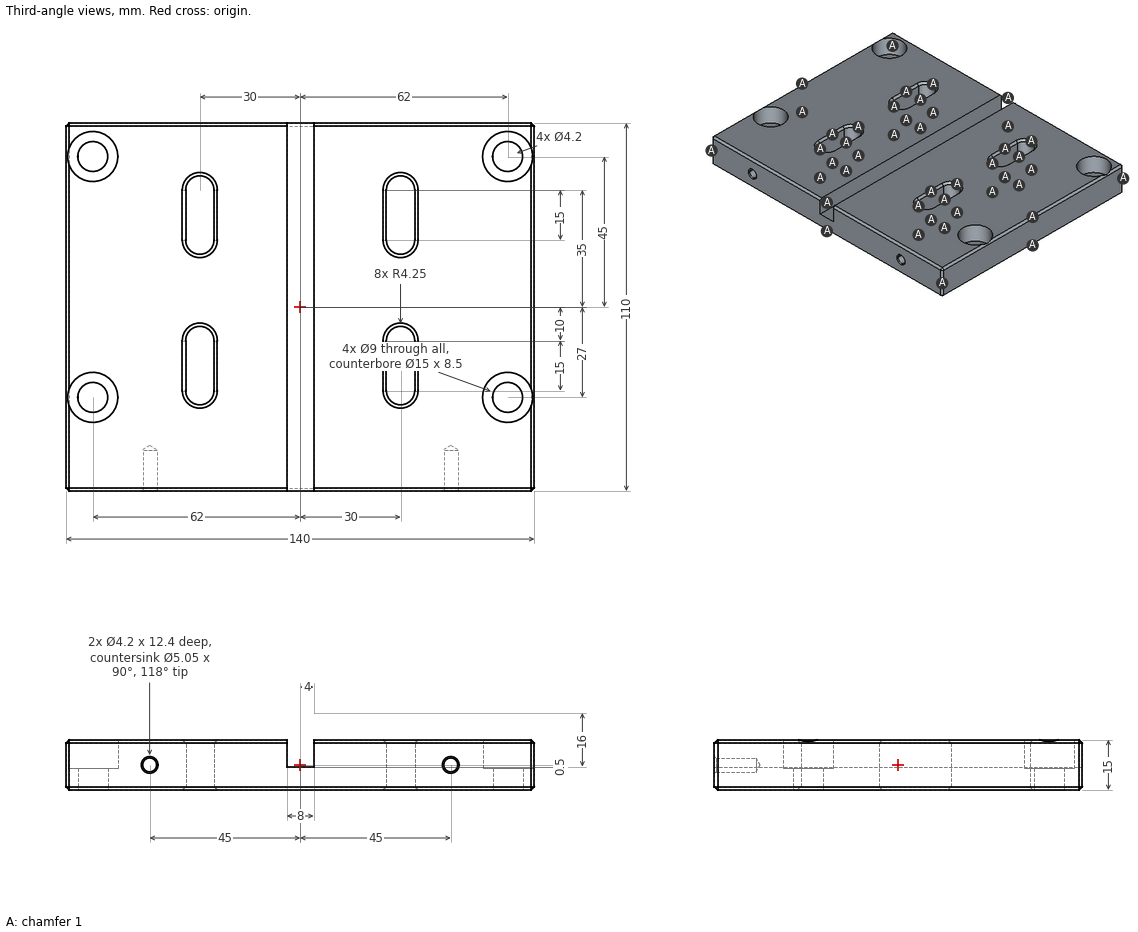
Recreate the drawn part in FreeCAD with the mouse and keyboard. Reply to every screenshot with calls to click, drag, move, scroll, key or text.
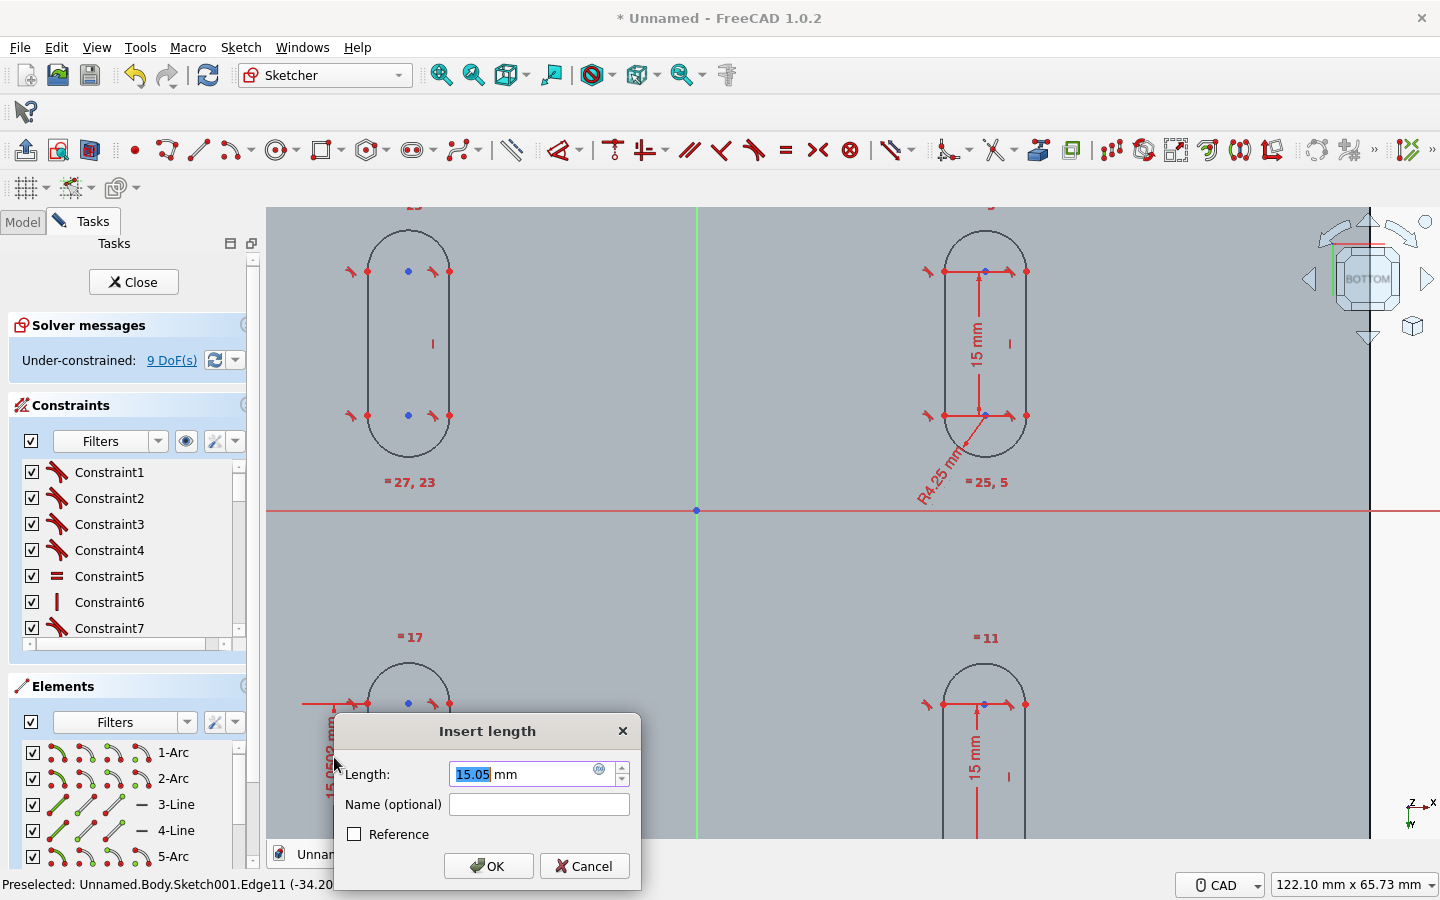
text(15)
key(Return)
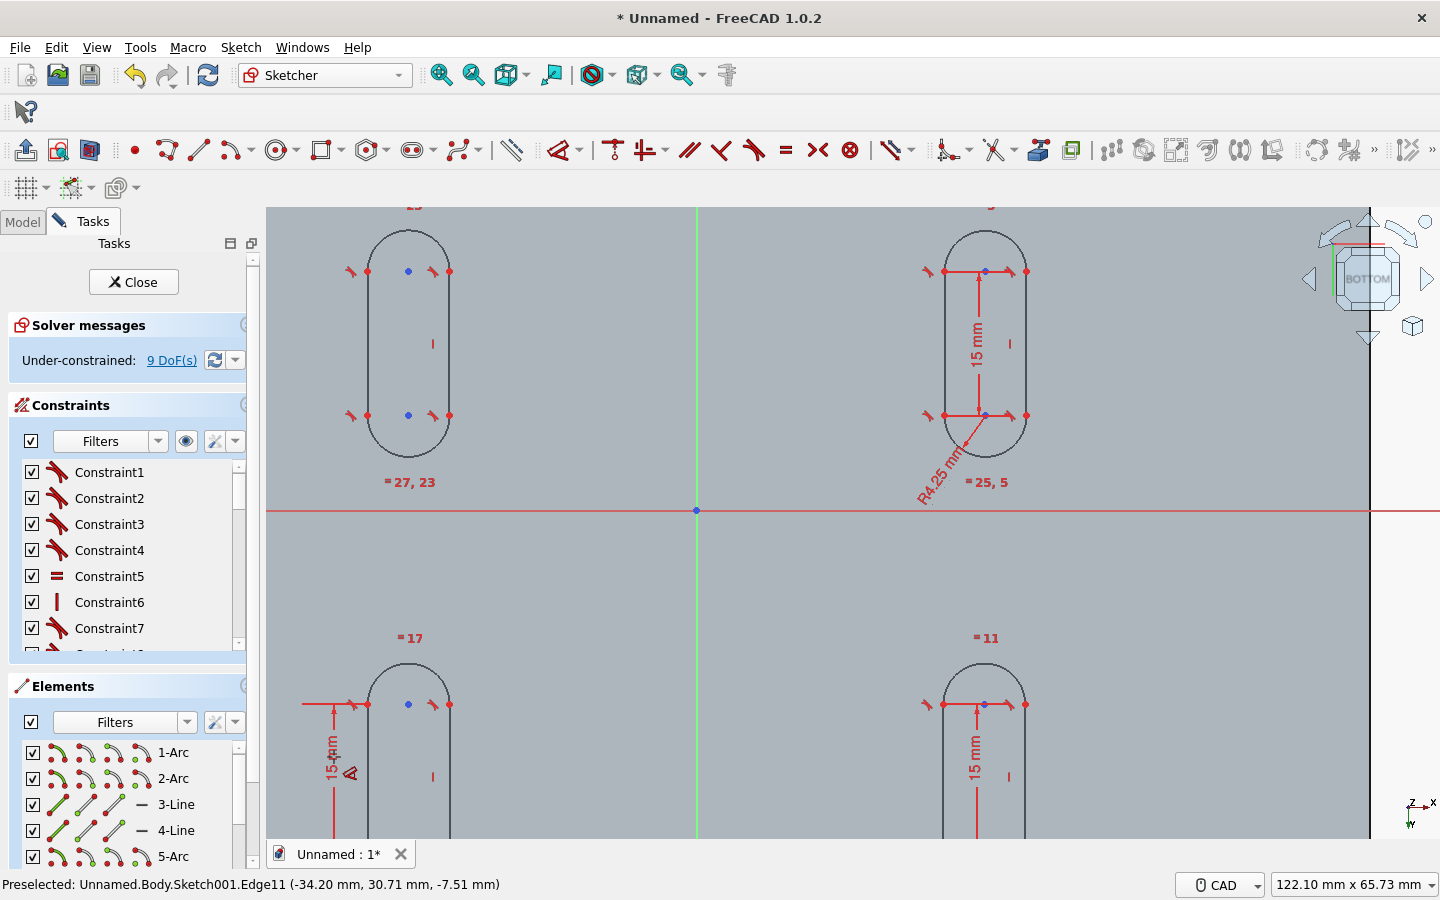
click(368, 373)
click(334, 344)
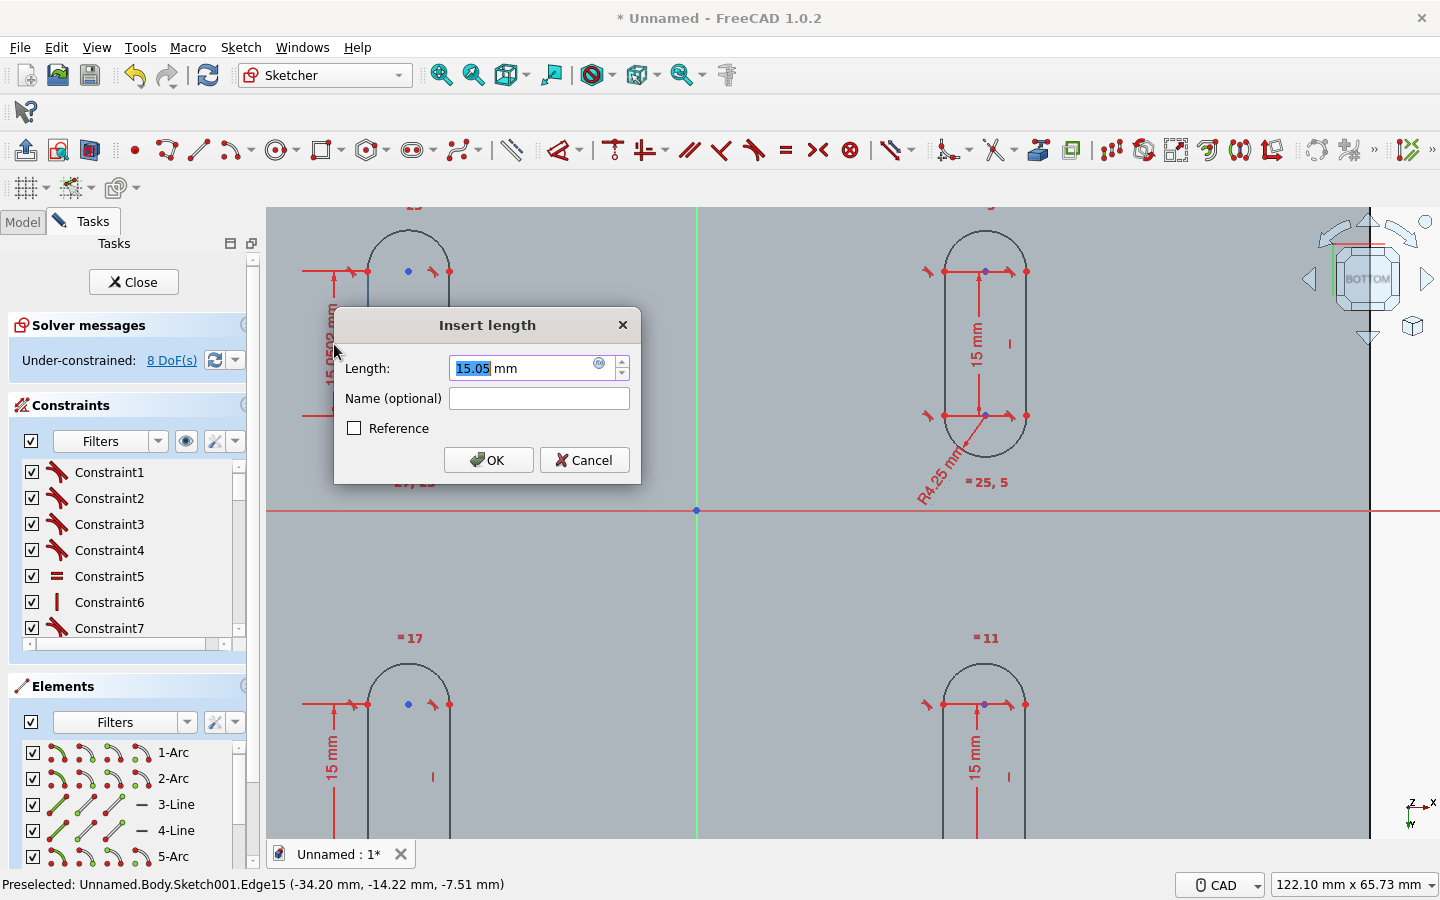
text(15)
key(Return)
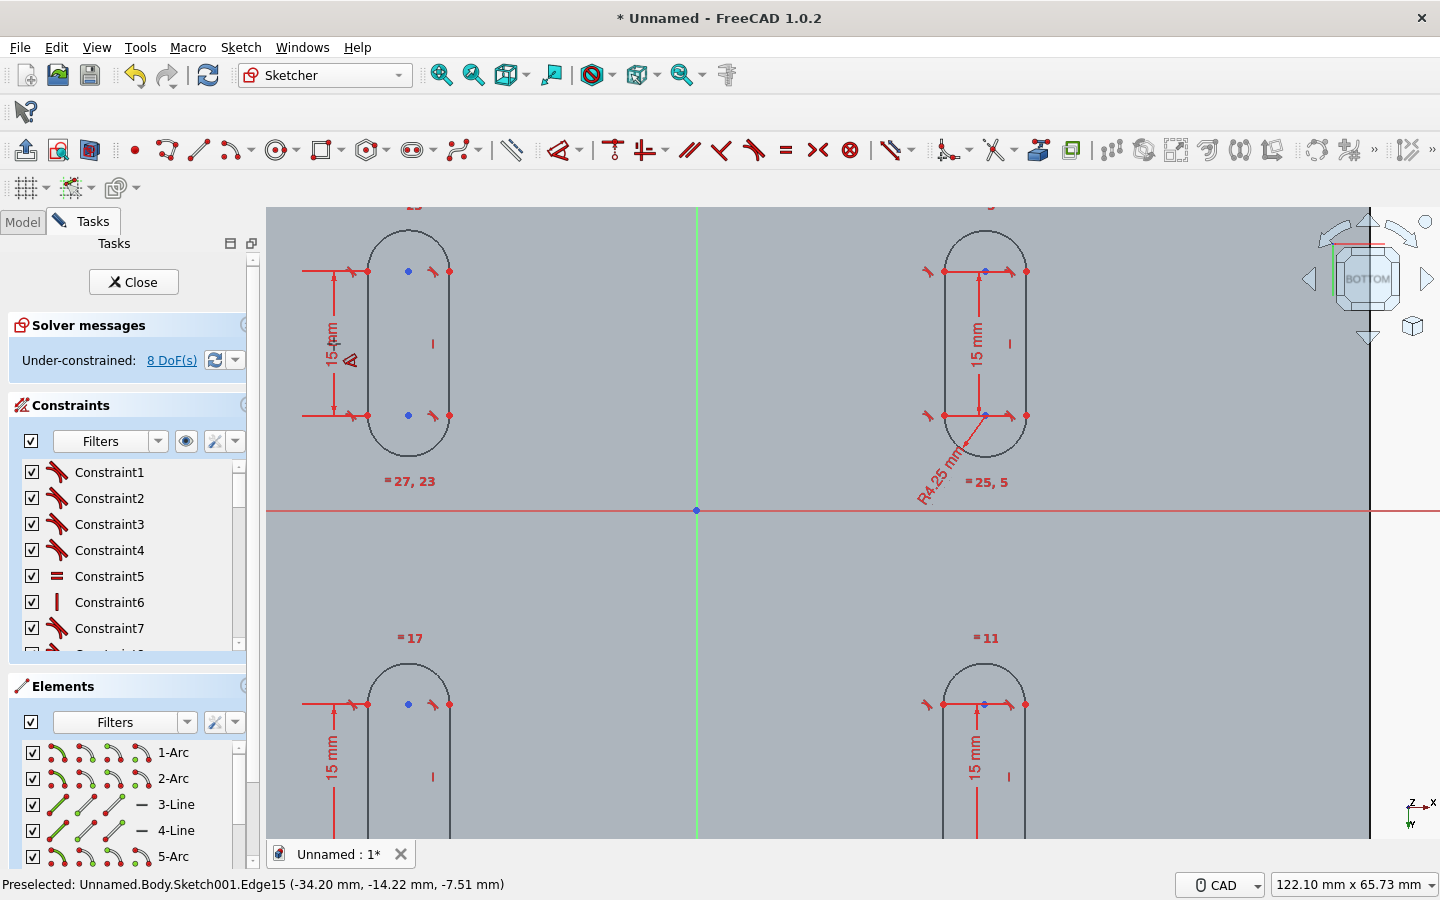
click(945, 416)
click(979, 442)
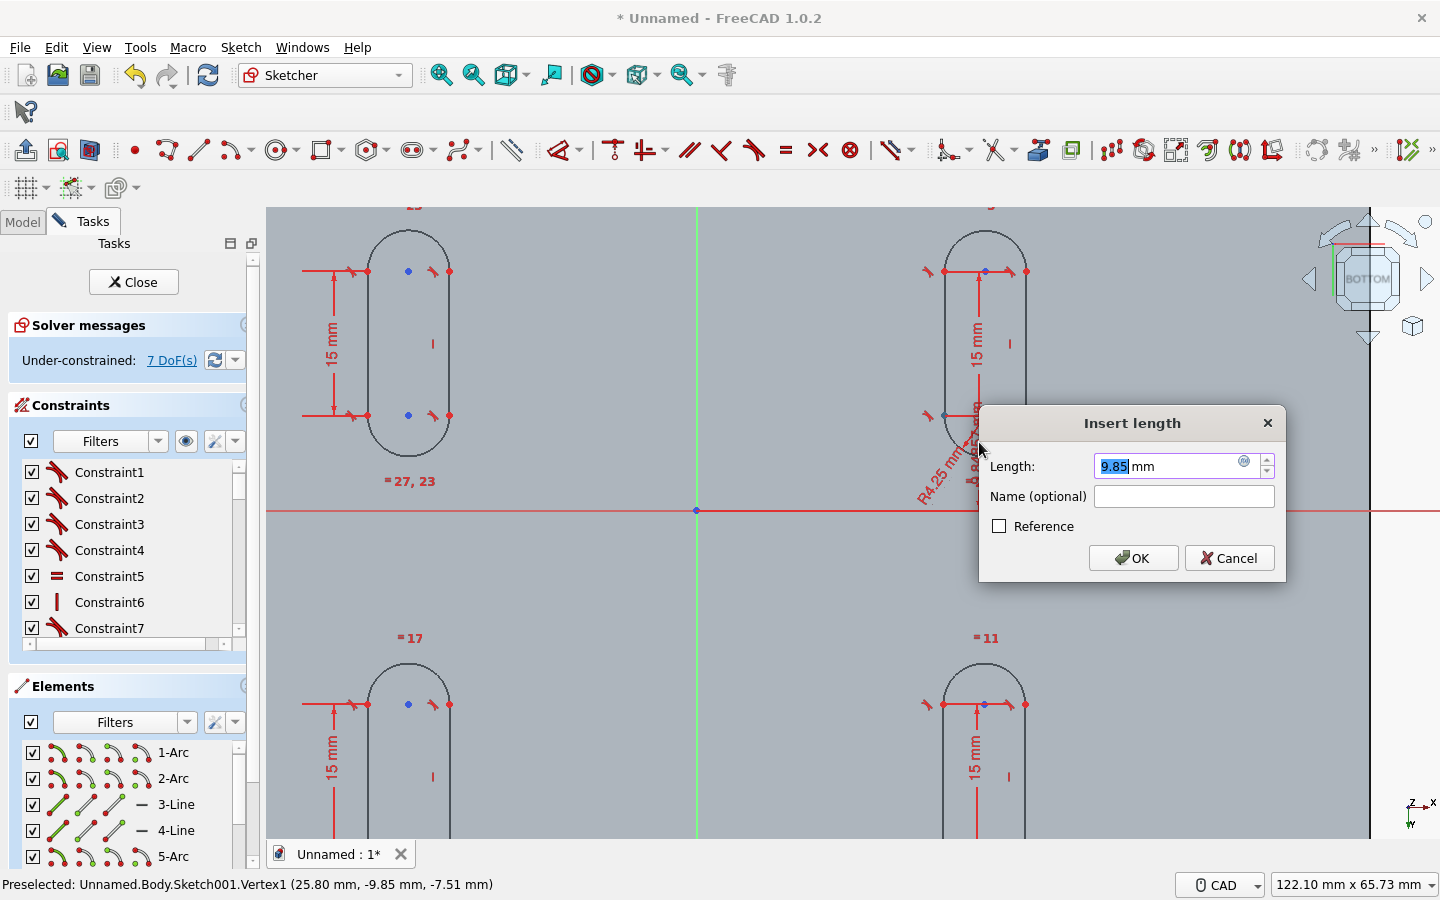
text(10)
key(Return)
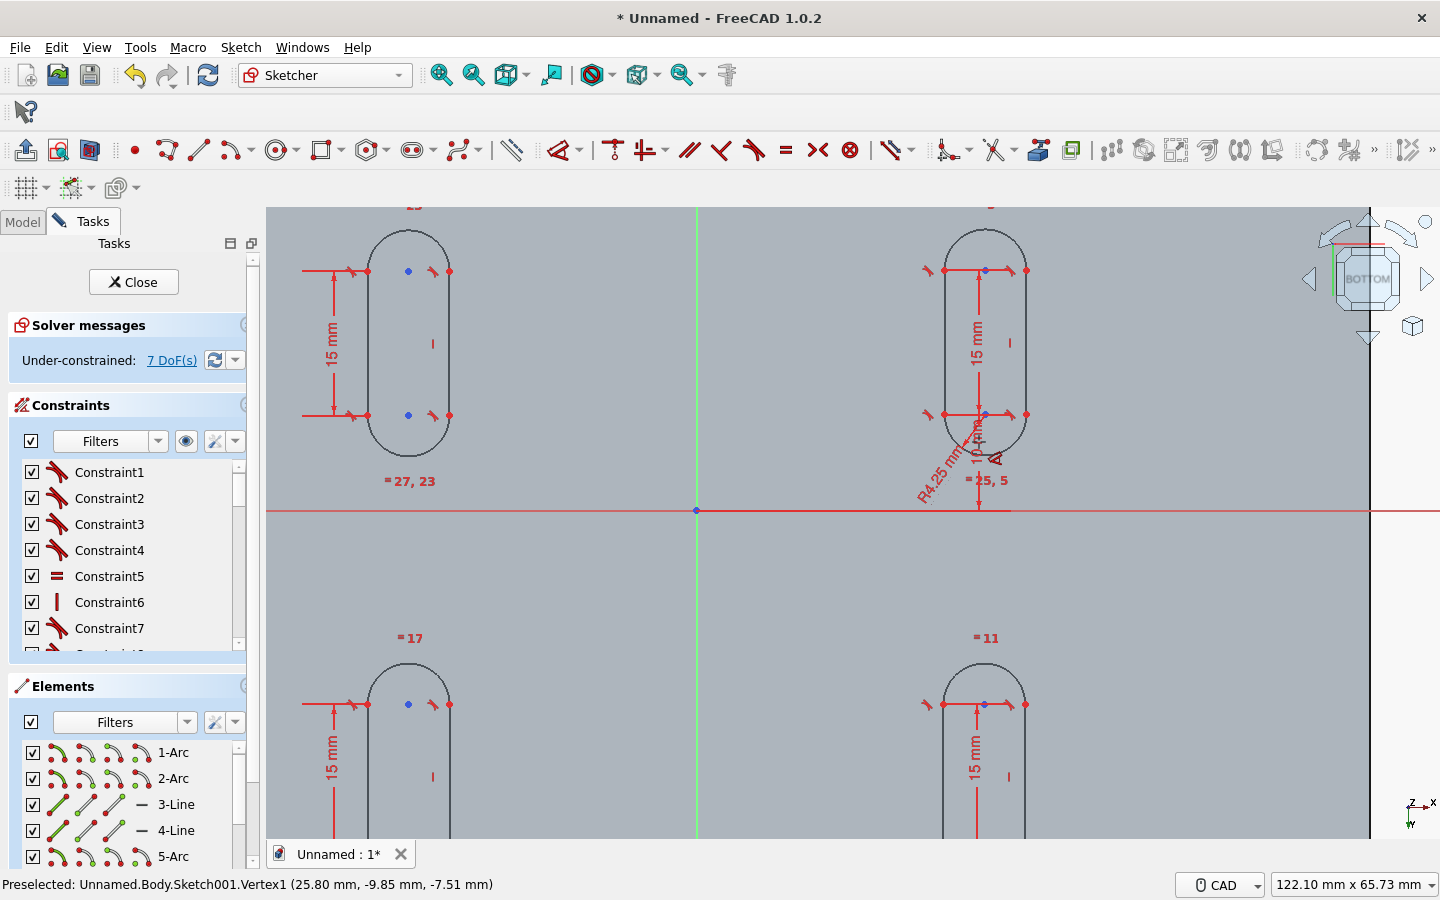
scroll(963, 450, down, 2)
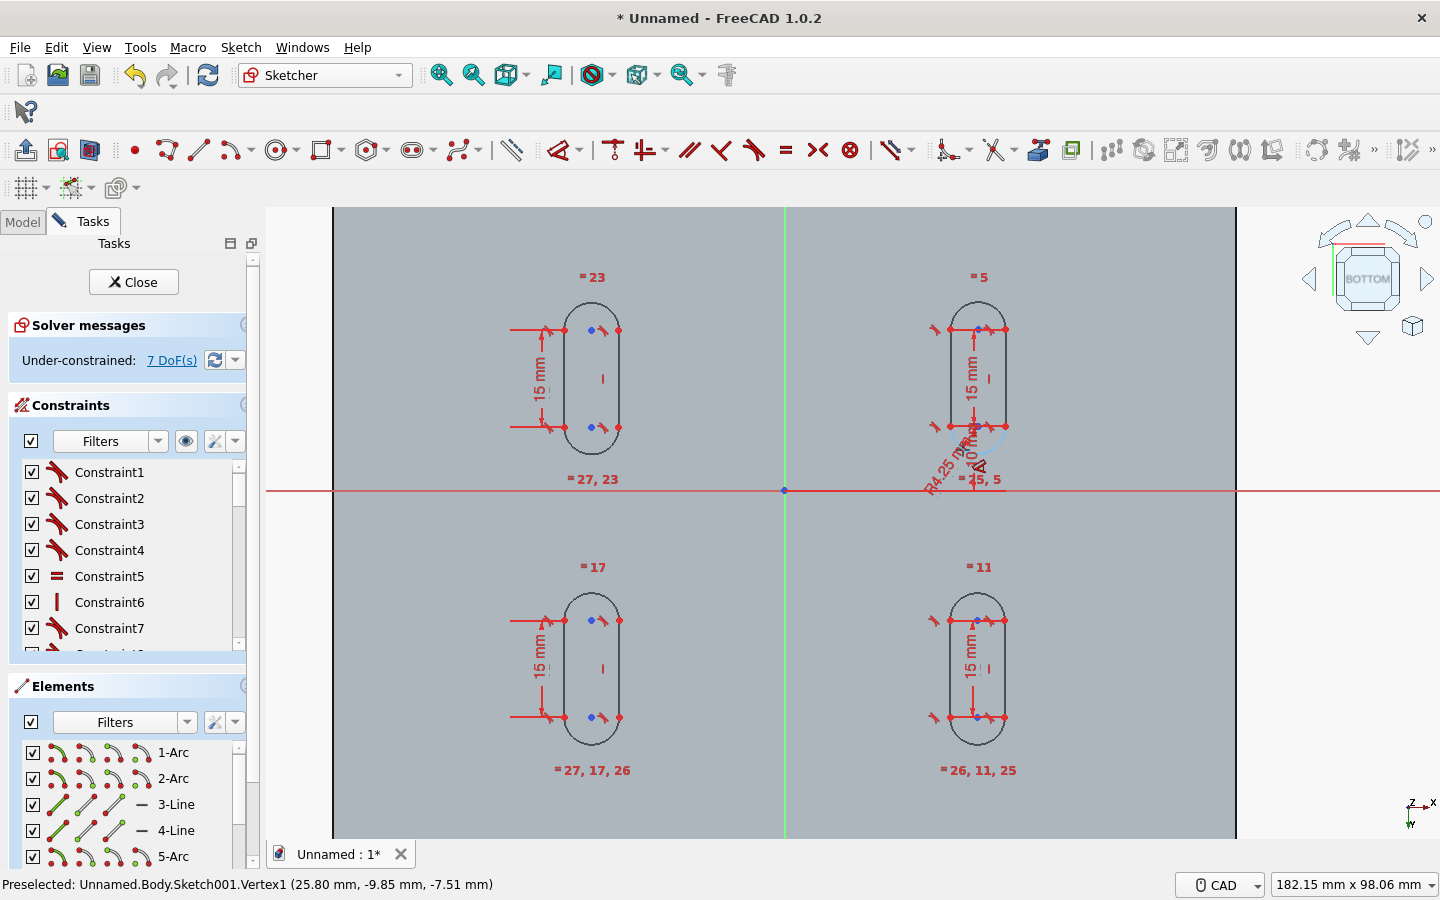
click(950, 717)
click(984, 552)